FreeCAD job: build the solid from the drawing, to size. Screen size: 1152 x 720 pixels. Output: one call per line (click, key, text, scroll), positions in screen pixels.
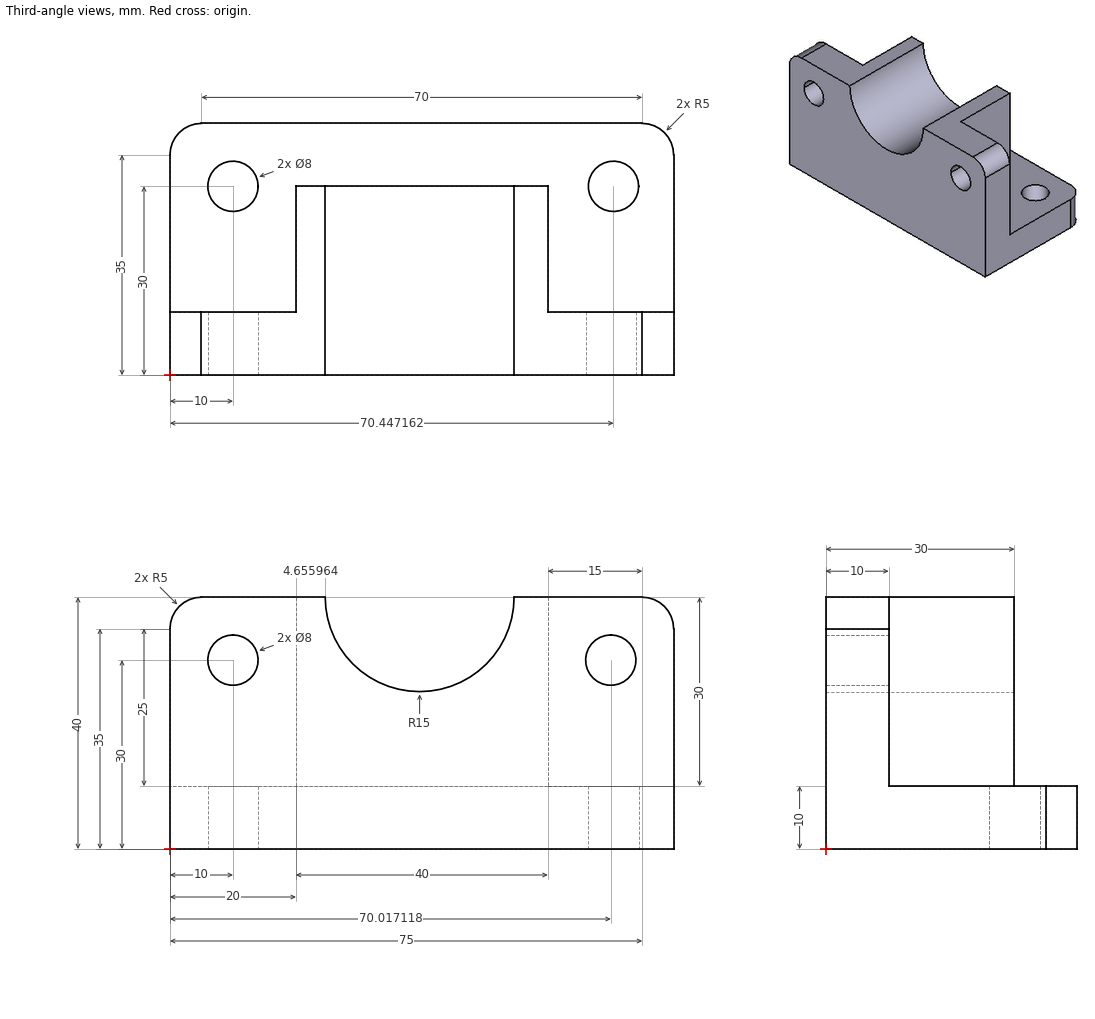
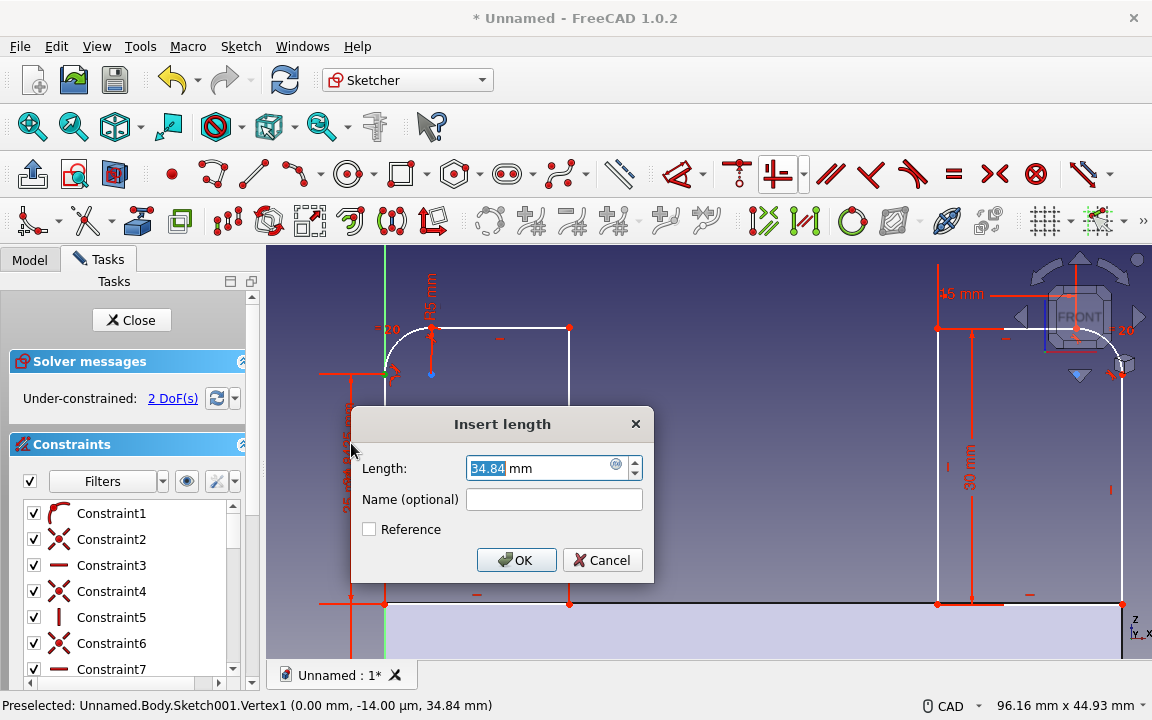
text(35)
key(Return)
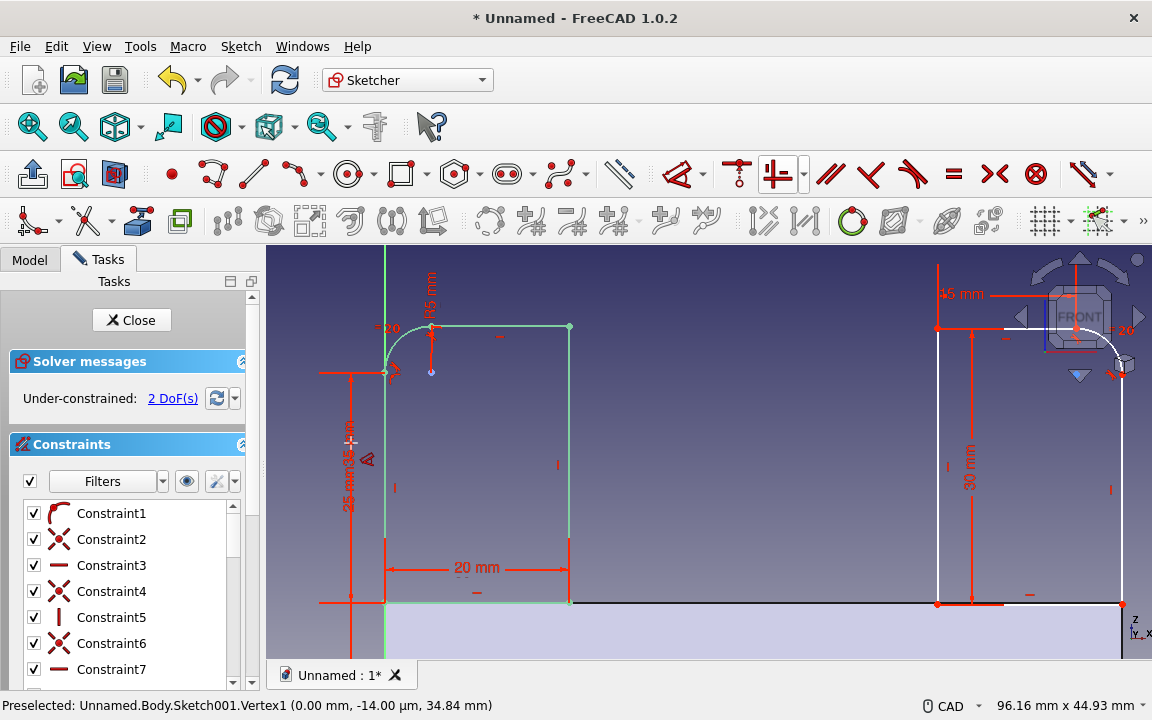
scroll(411, 333, down, 2)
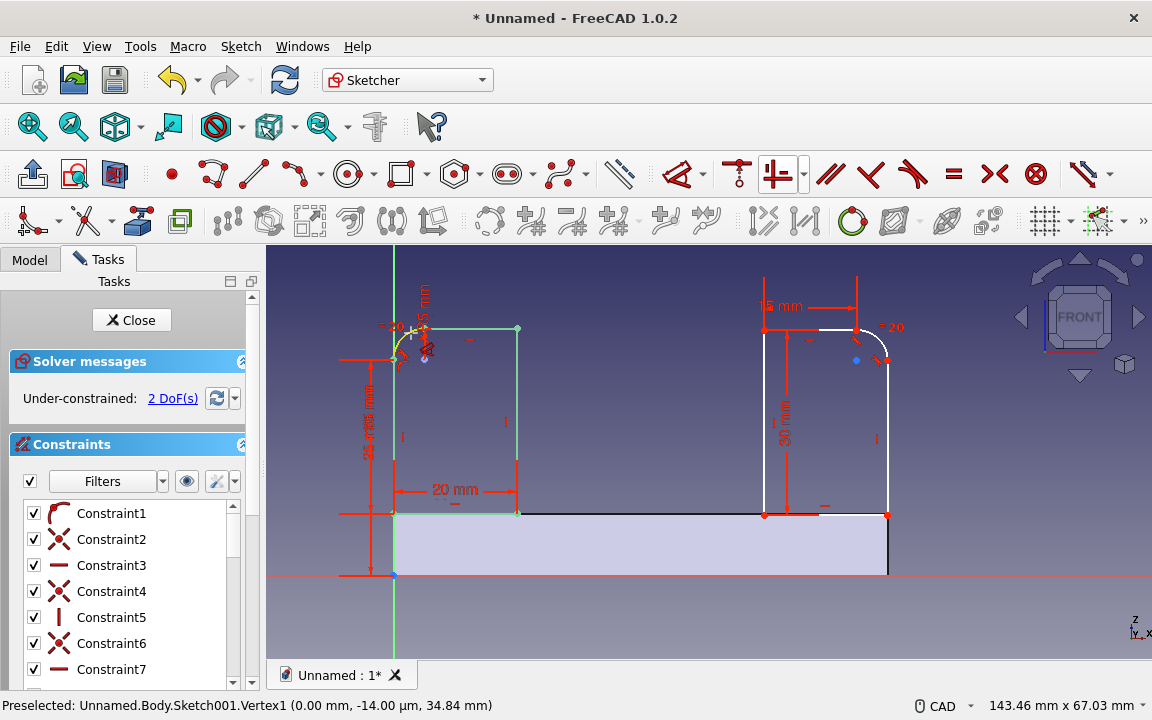
click(857, 330)
click(625, 610)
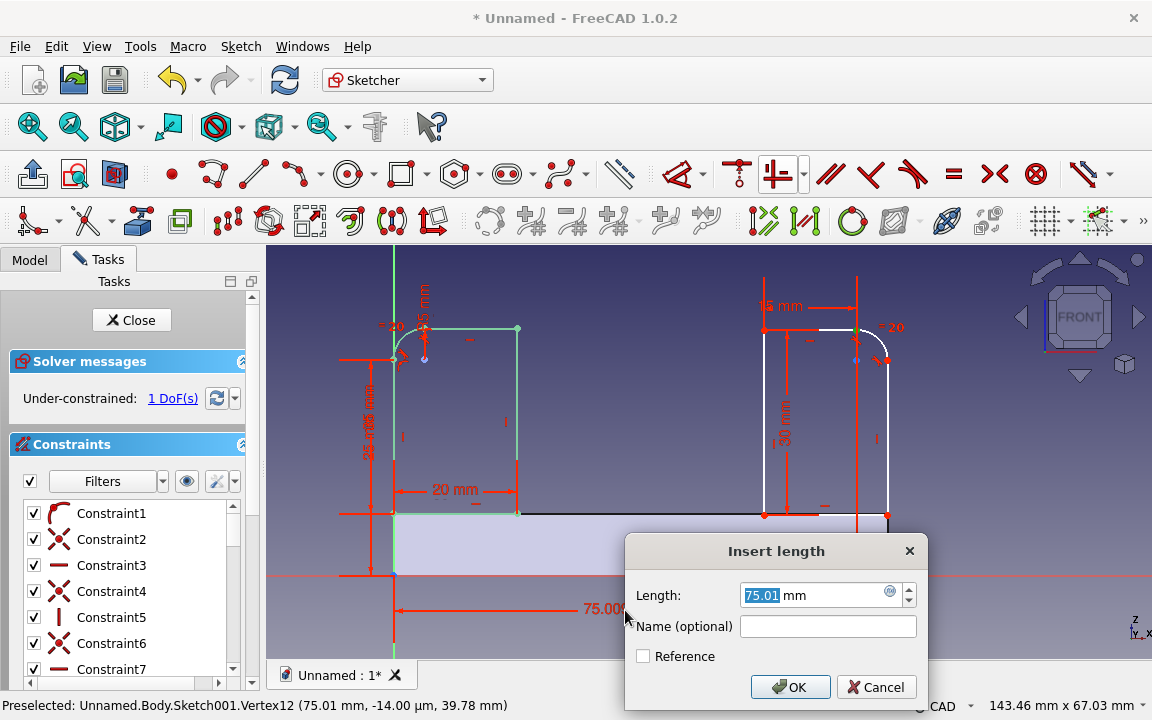
text(75)
key(Return)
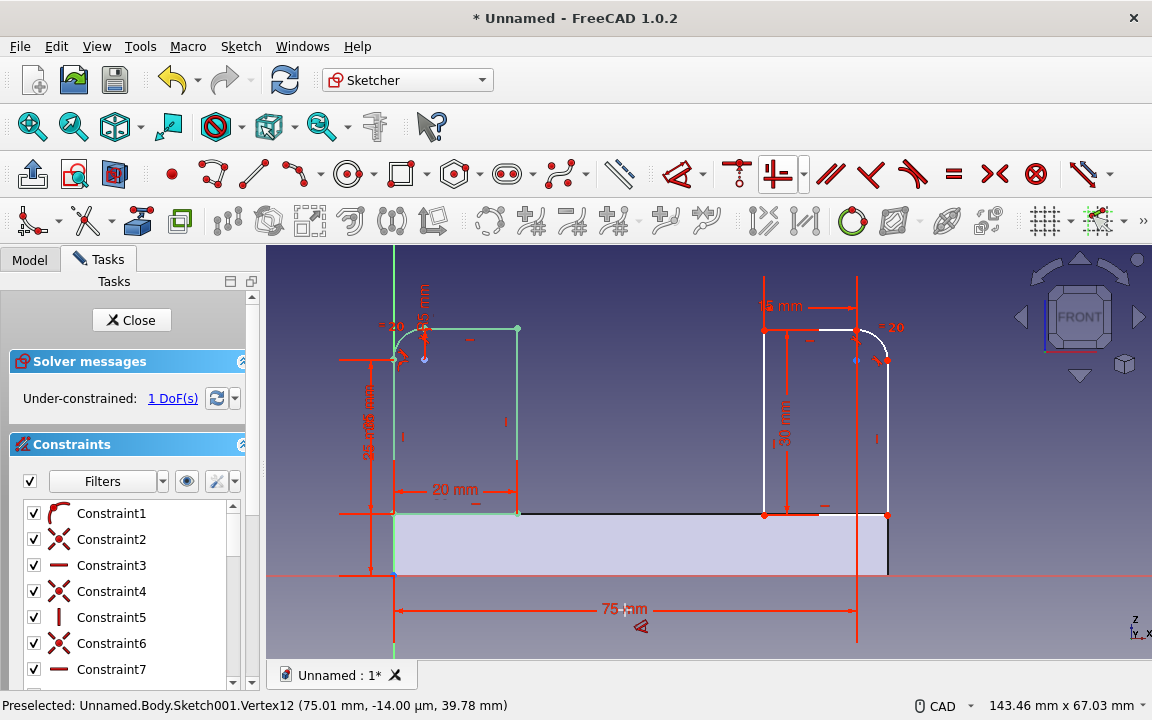
click(857, 330)
click(360, 509)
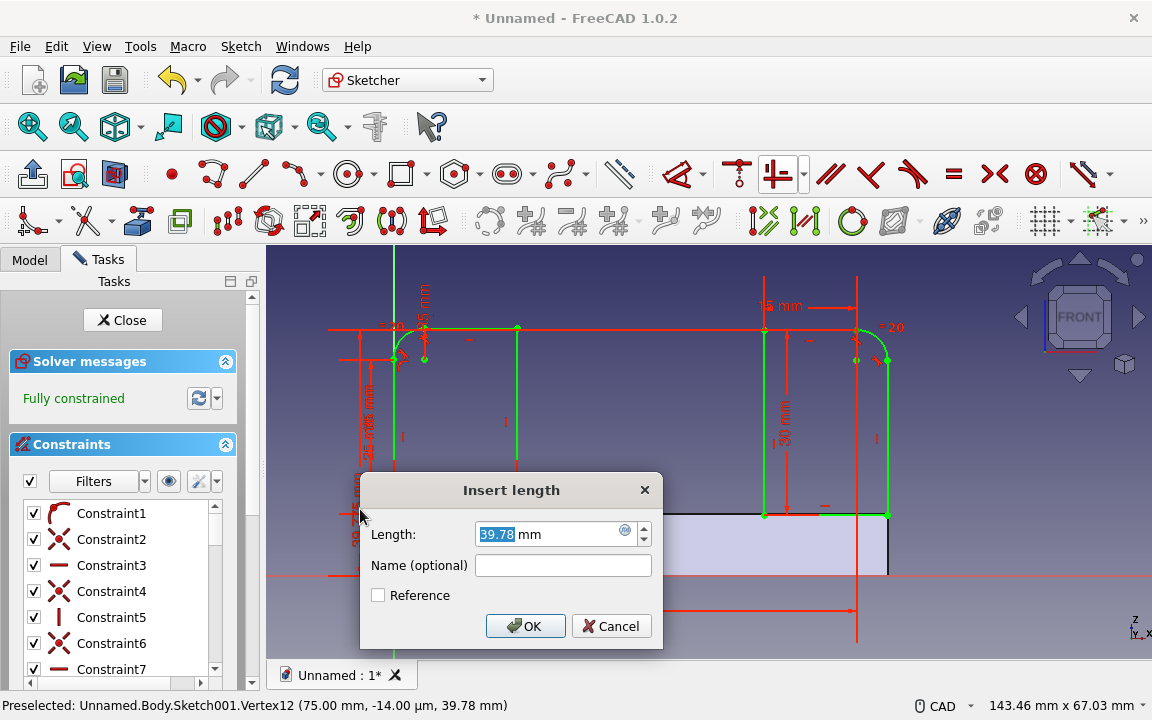
text(40)
key(Return)
key(Escape)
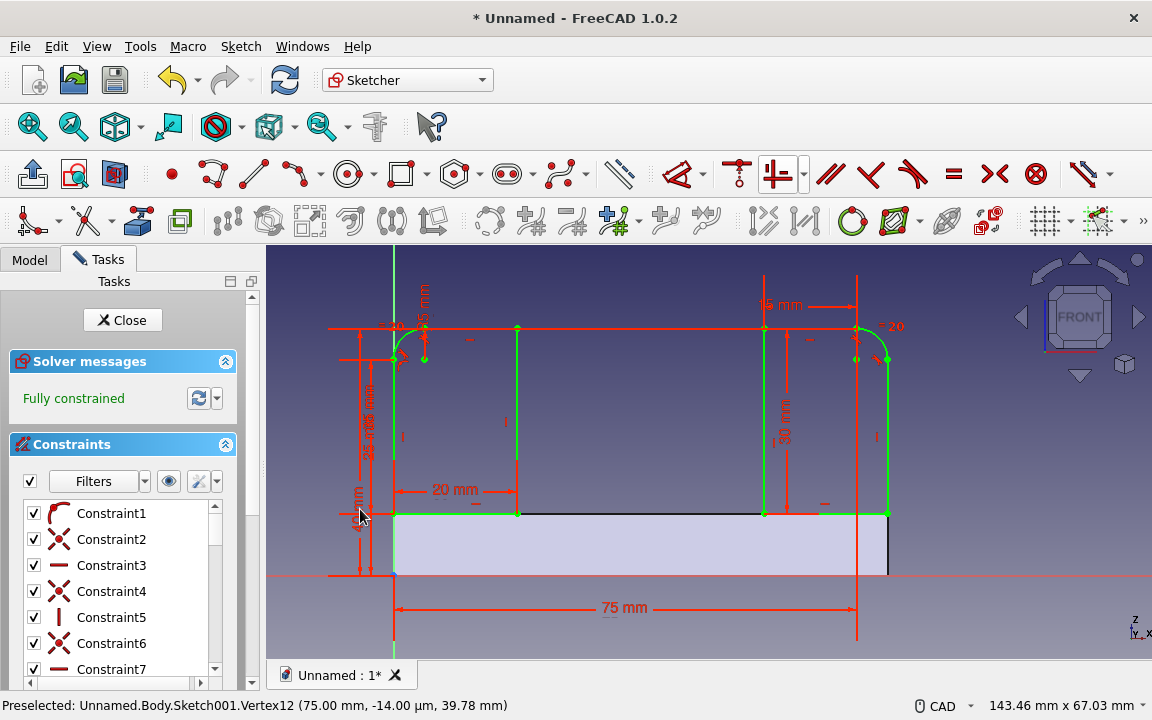
click(123, 320)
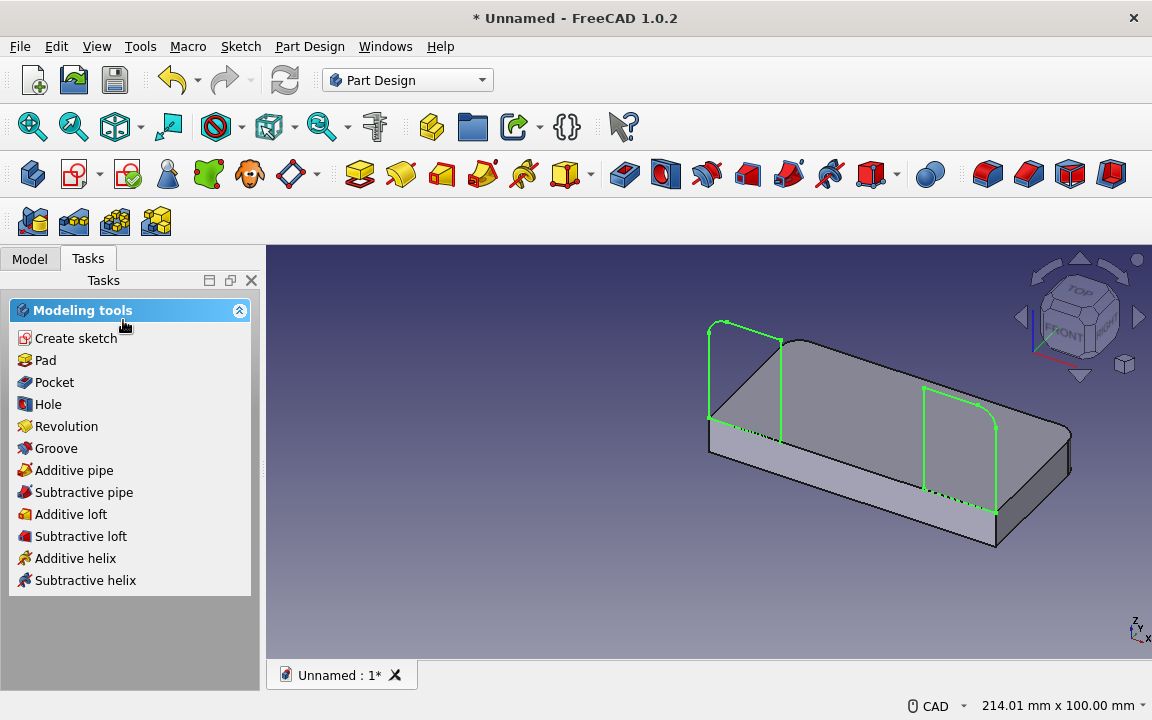
click(360, 174)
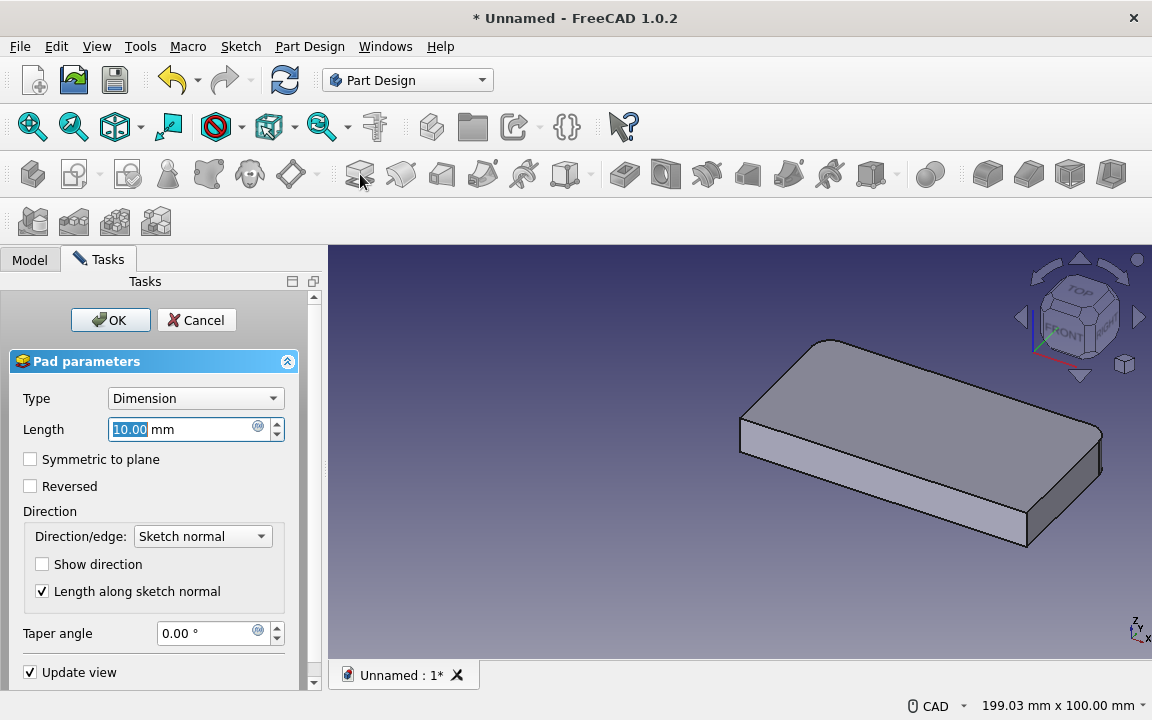
text(10)
key(Tab)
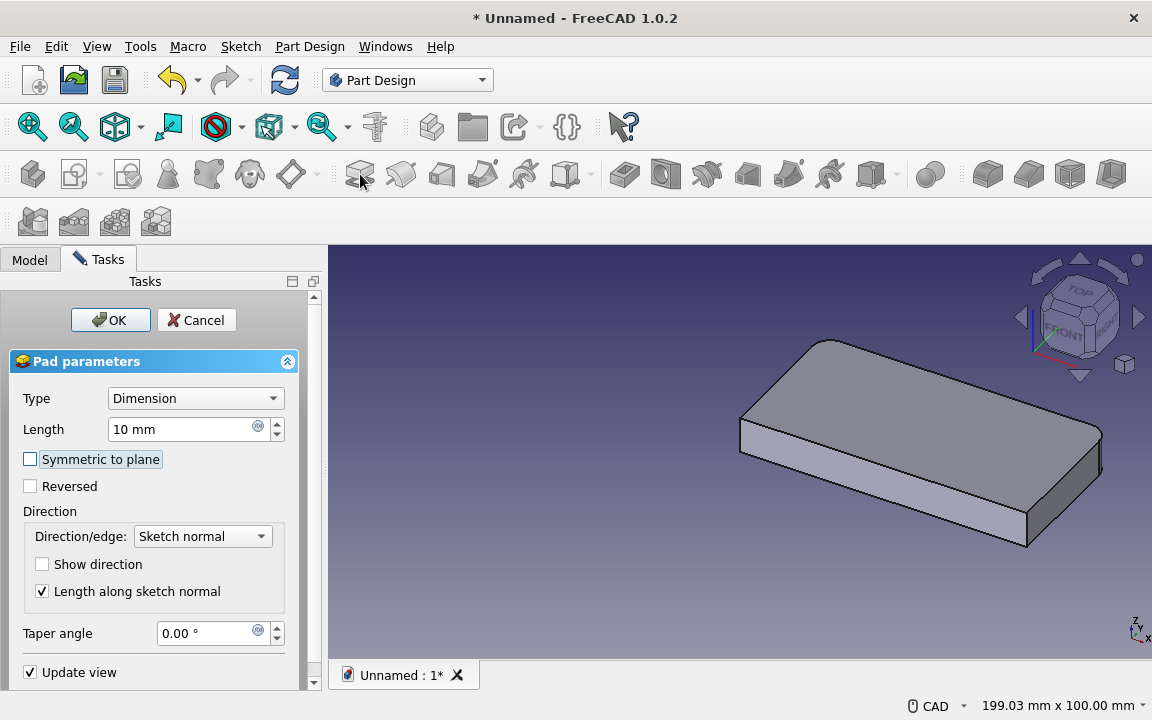
click(31, 486)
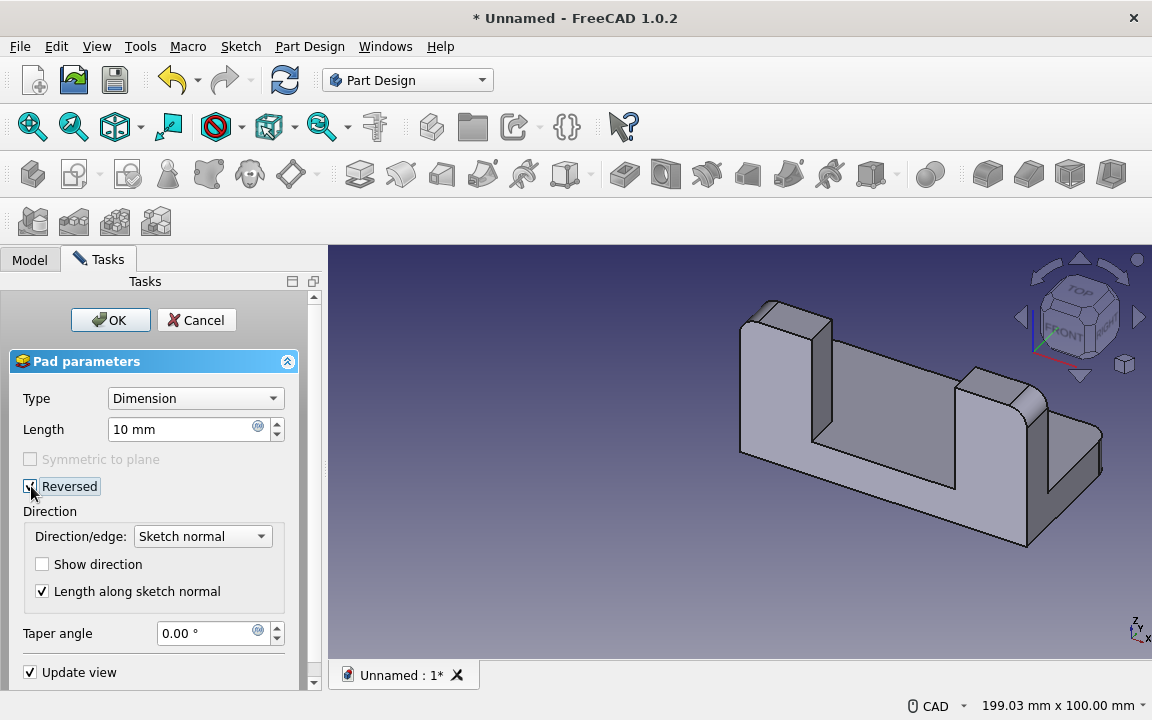
click(111, 320)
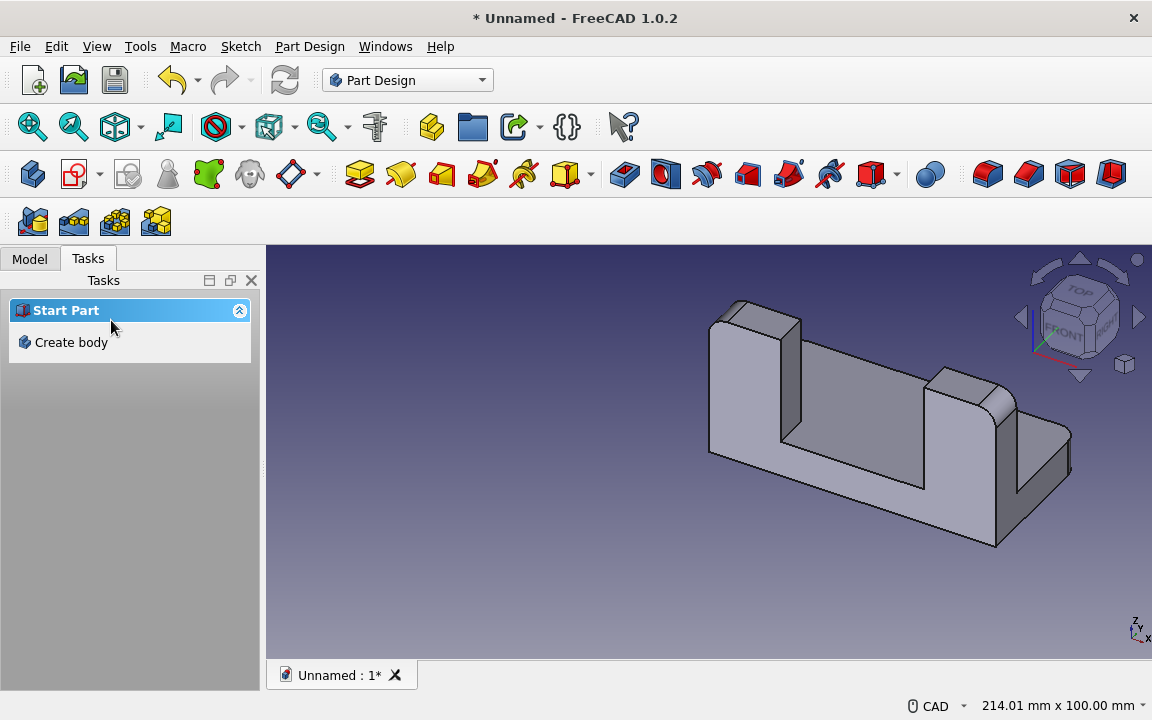
click(33, 128)